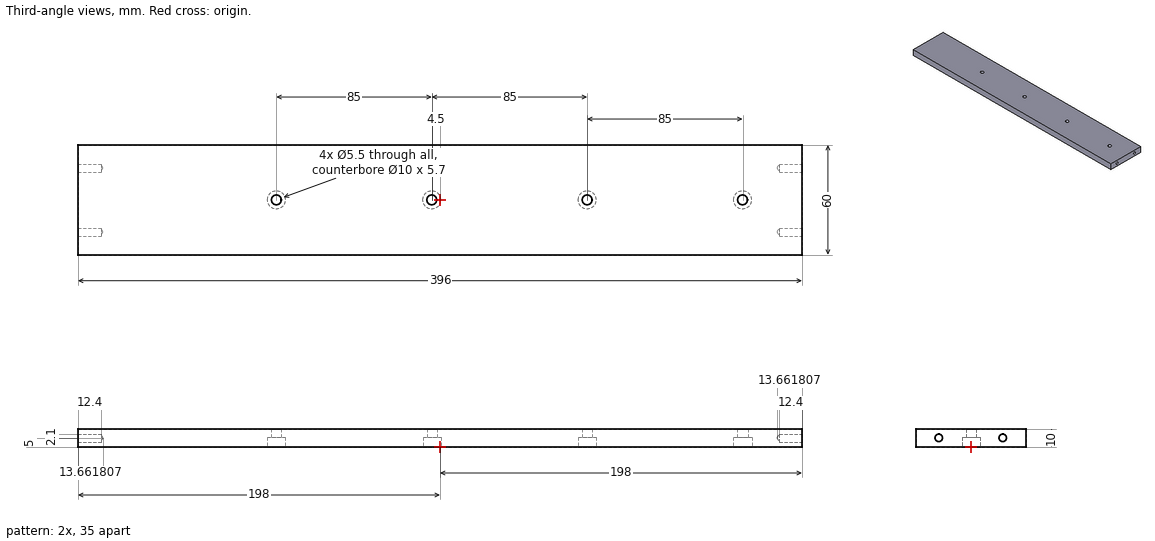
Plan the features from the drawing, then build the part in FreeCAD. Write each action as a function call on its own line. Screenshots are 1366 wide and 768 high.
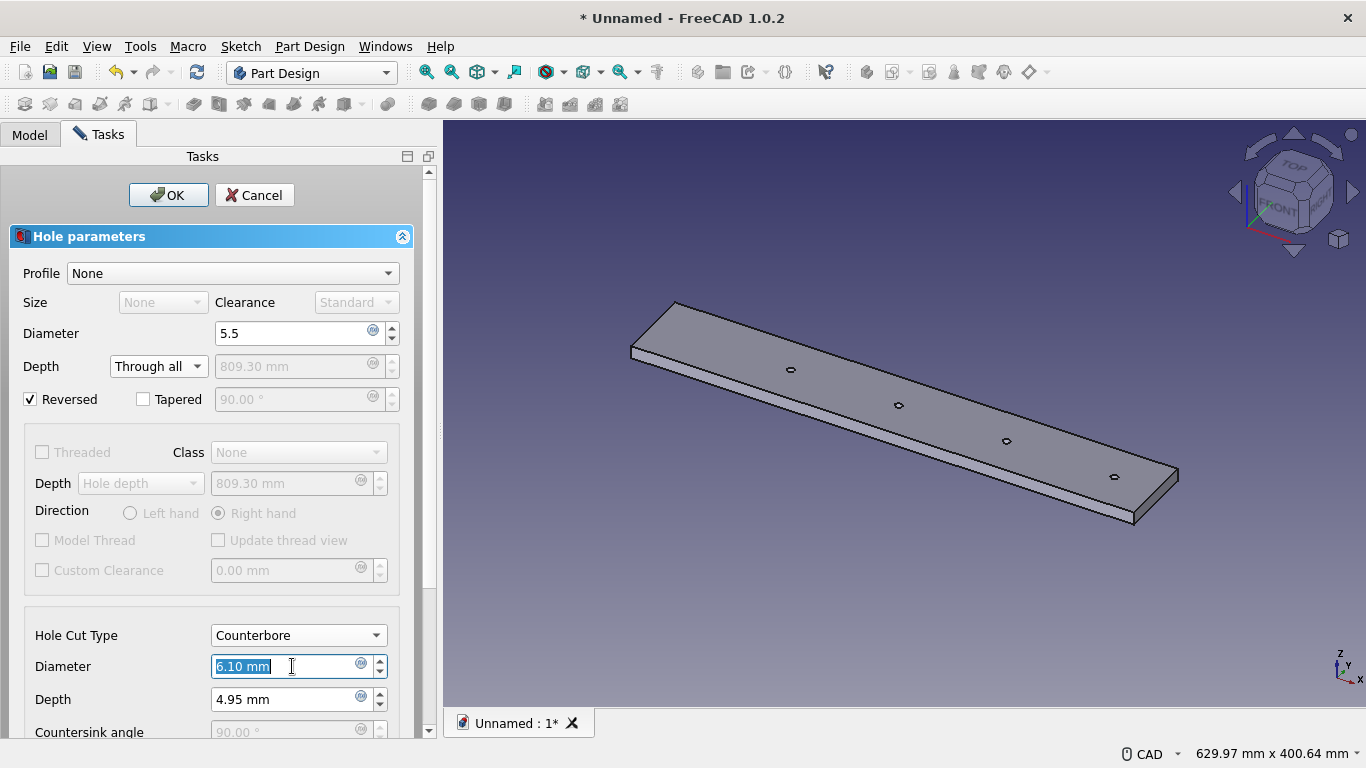
text(10)
key(Tab)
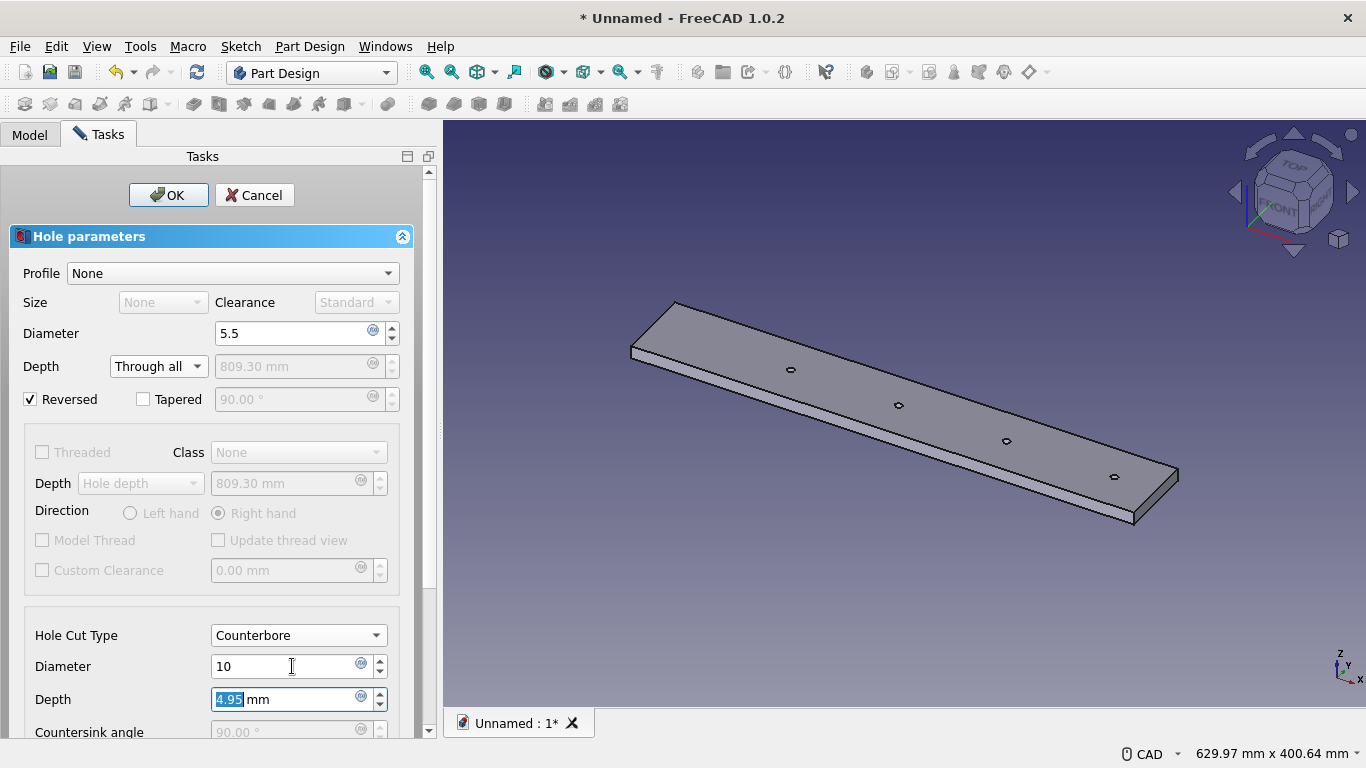
text(5.7)
key(Tab)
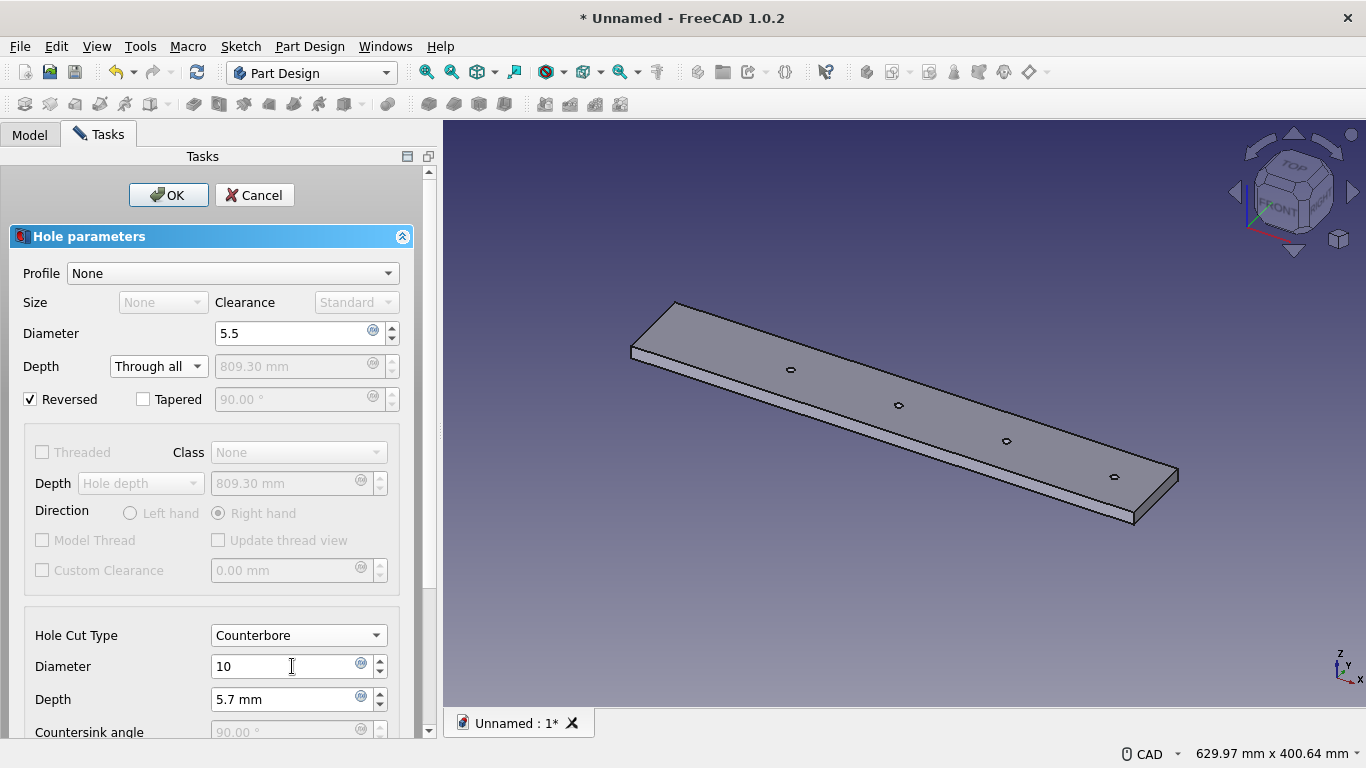
click(169, 195)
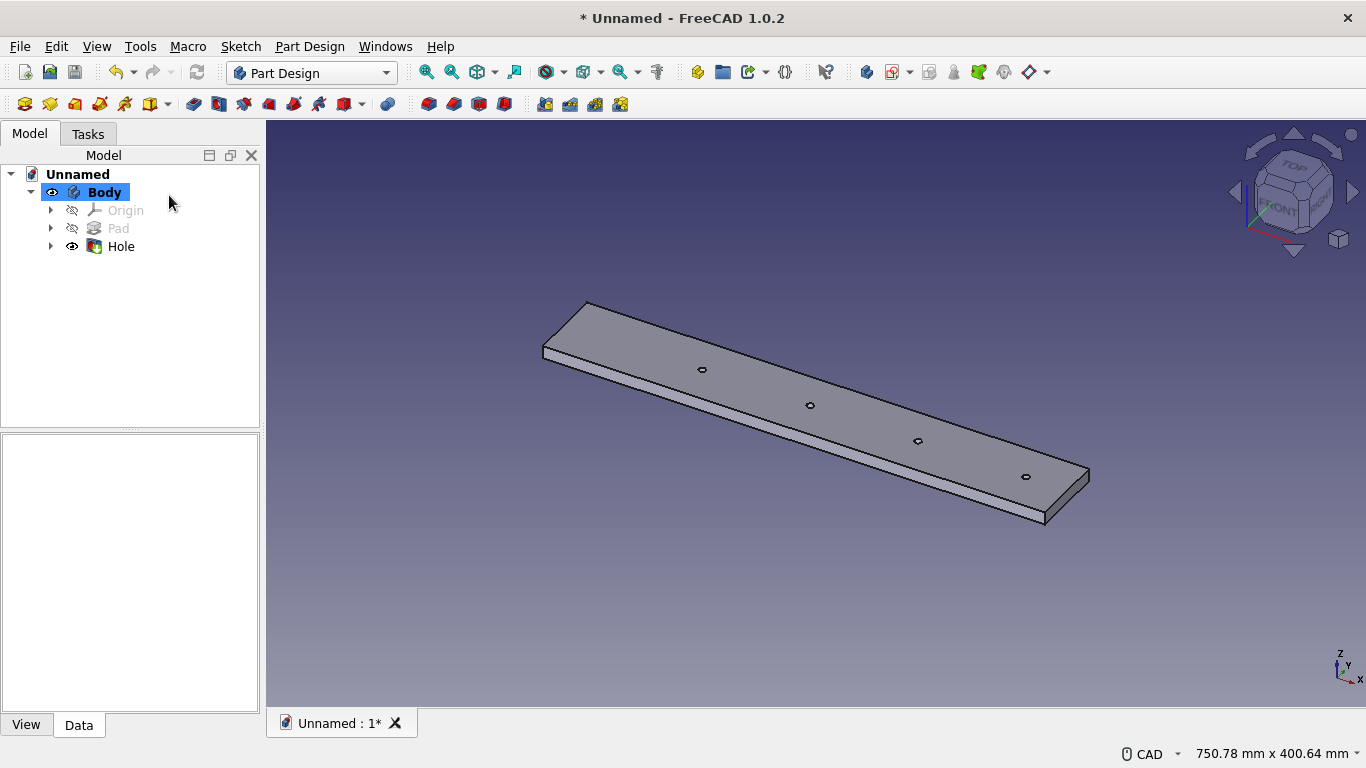
click(51, 210)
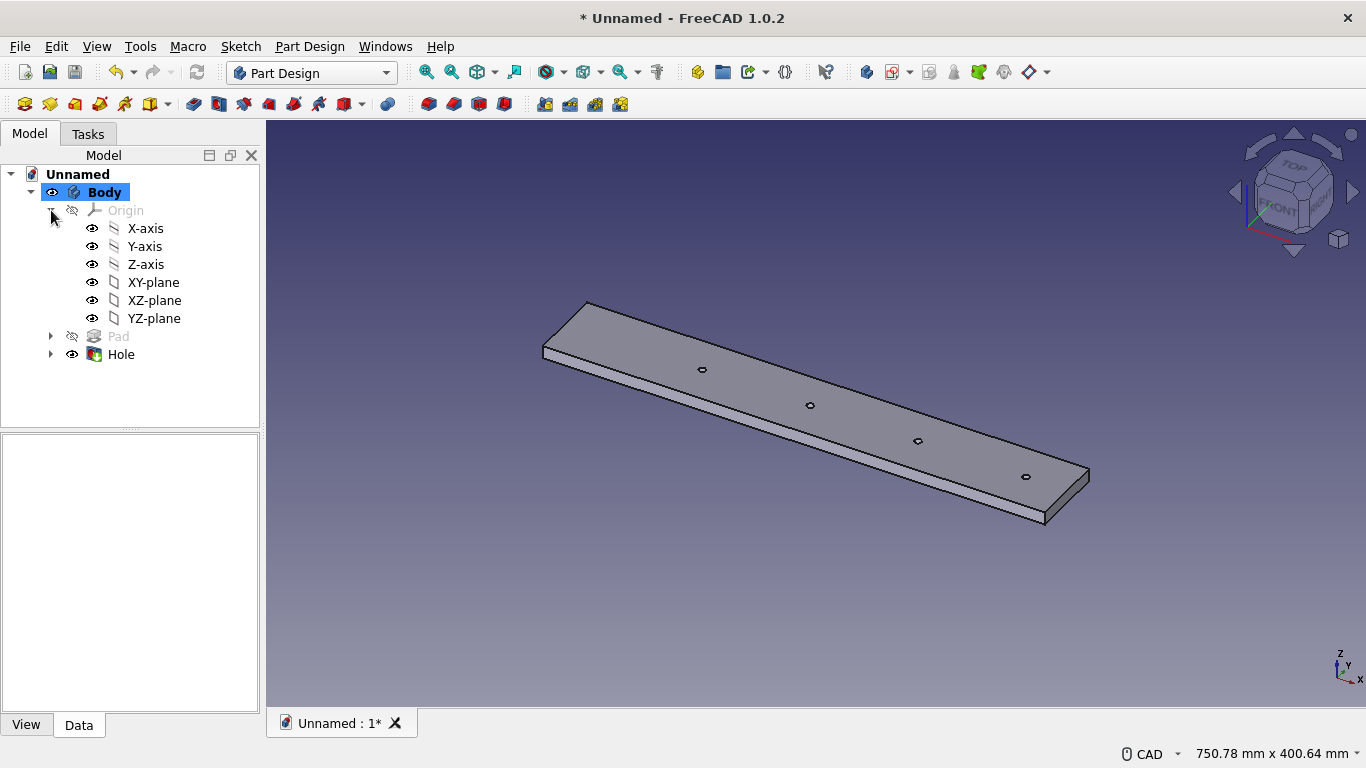
click(137, 300)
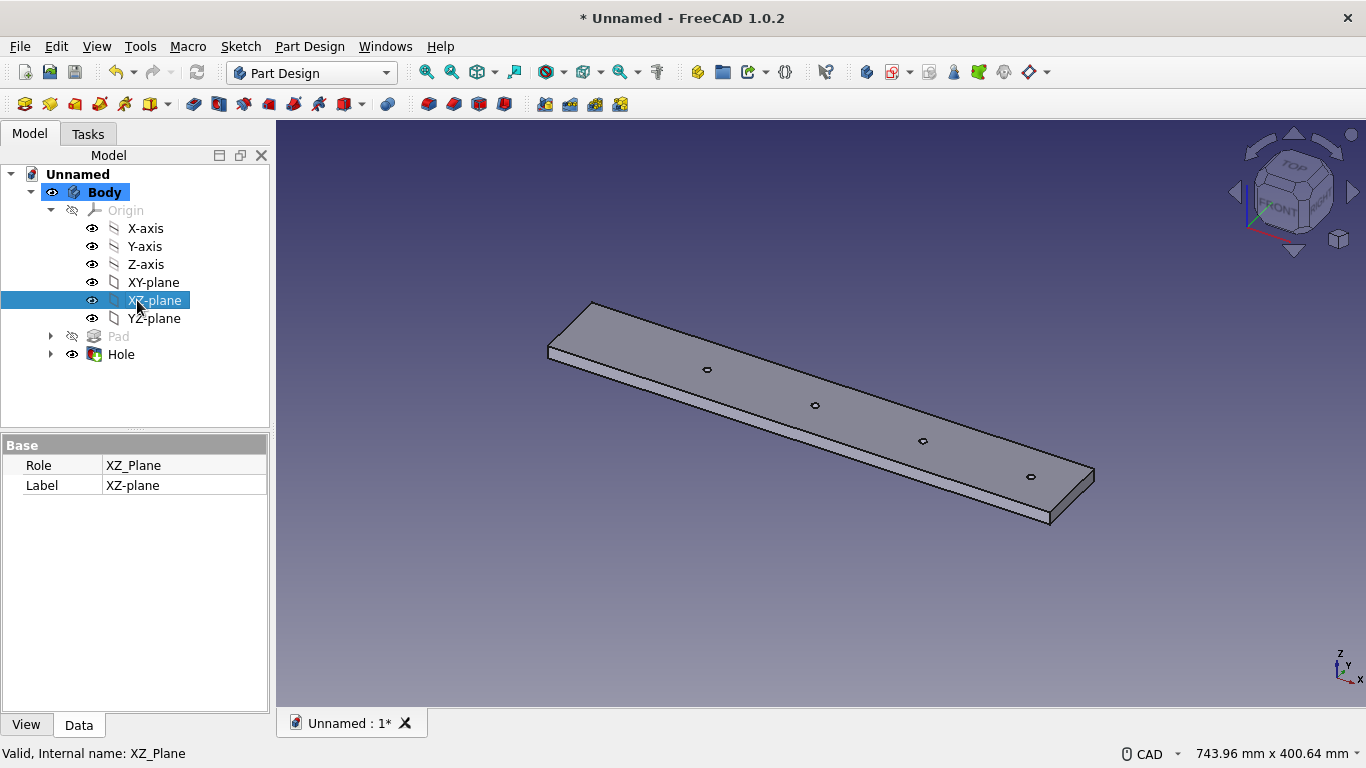
click(1028, 72)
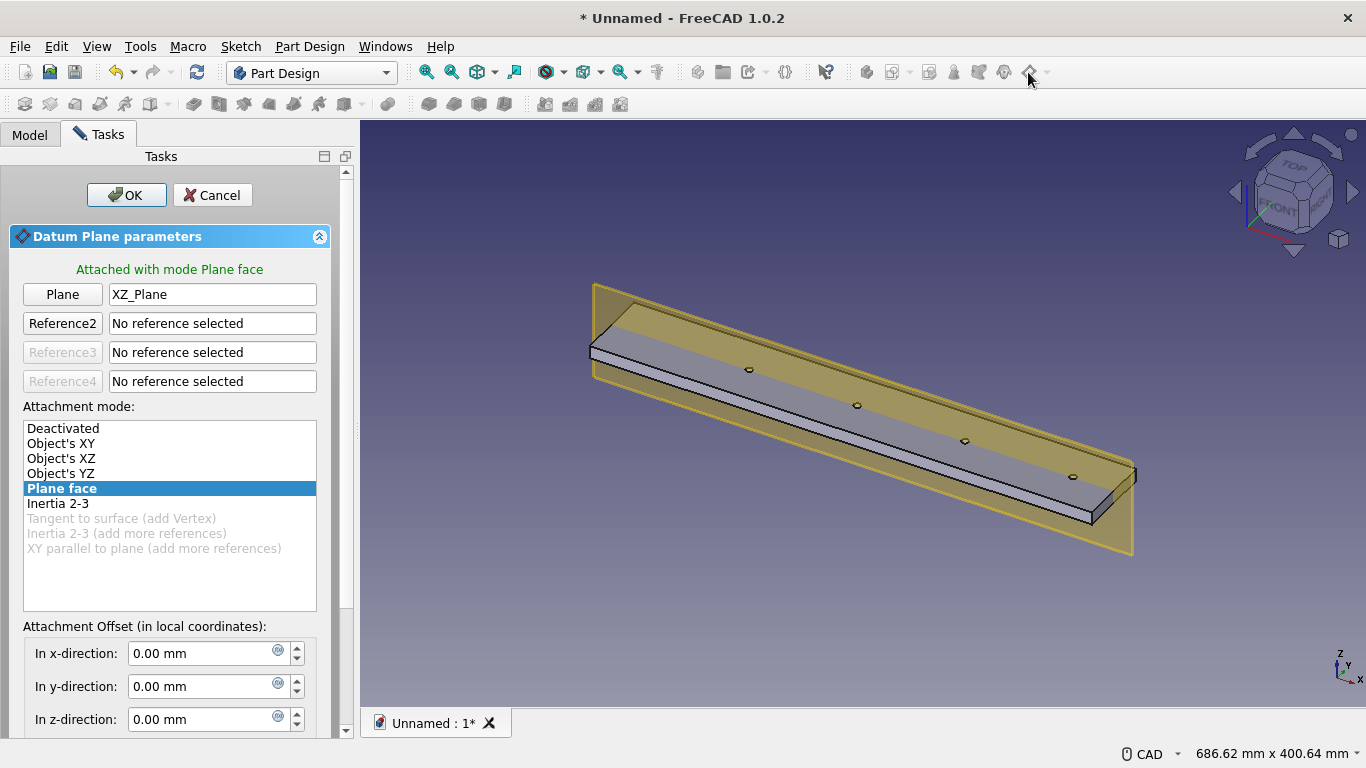
triple_click(210, 720)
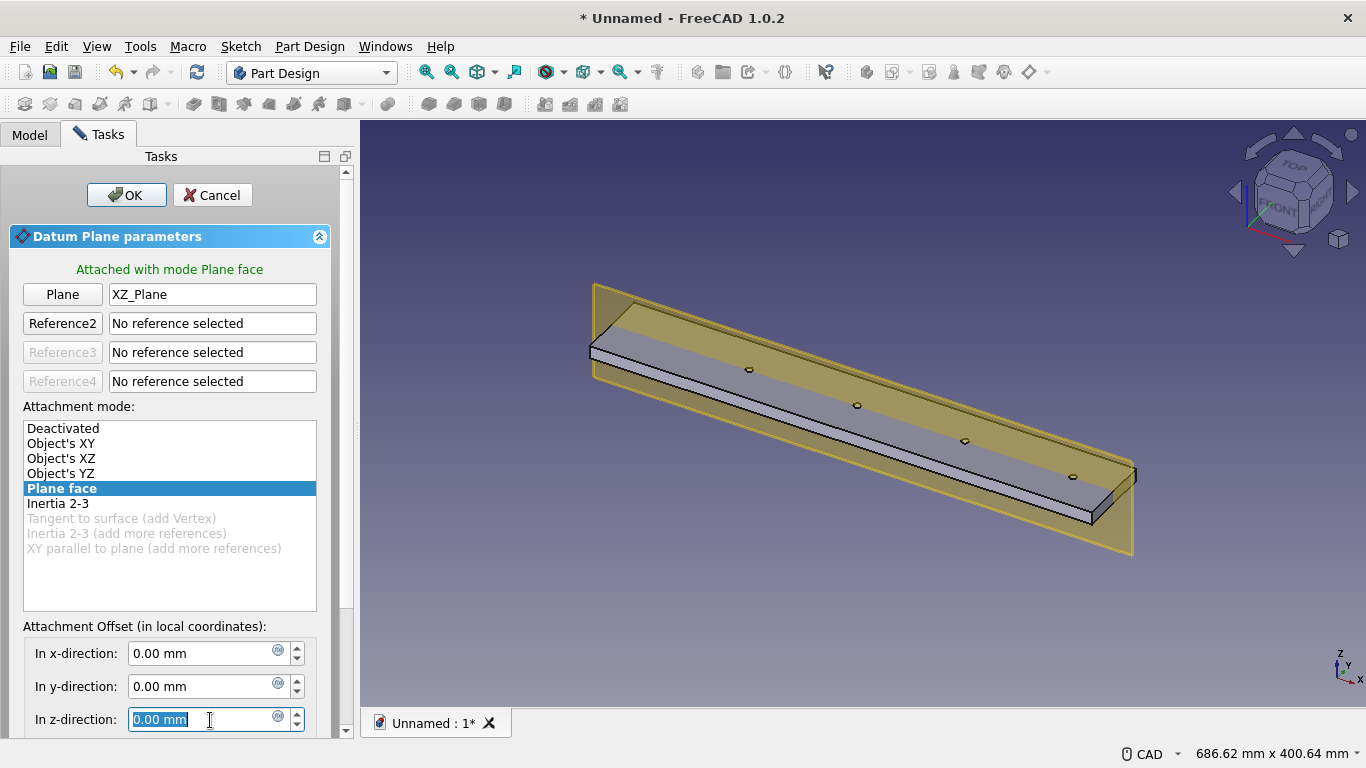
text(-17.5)
key(Tab)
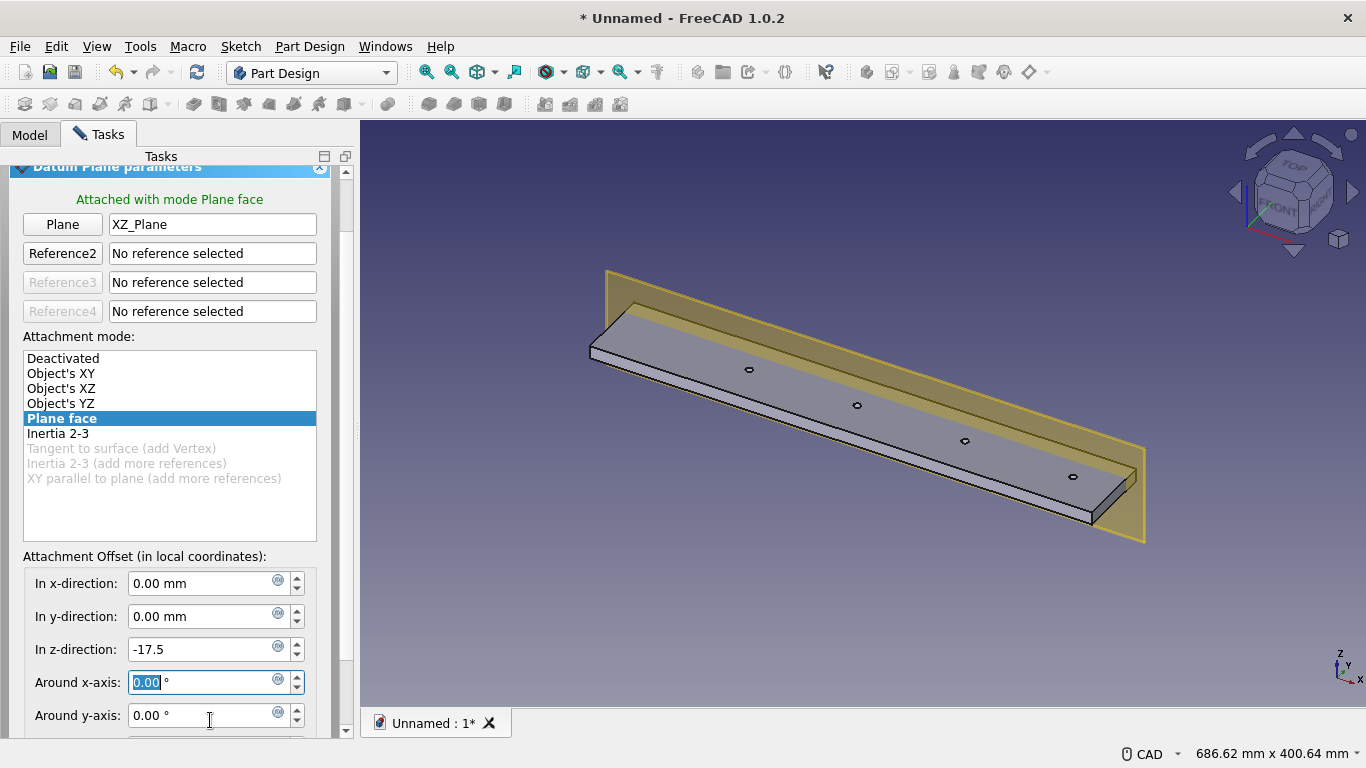
scroll(346, 452, up, 2)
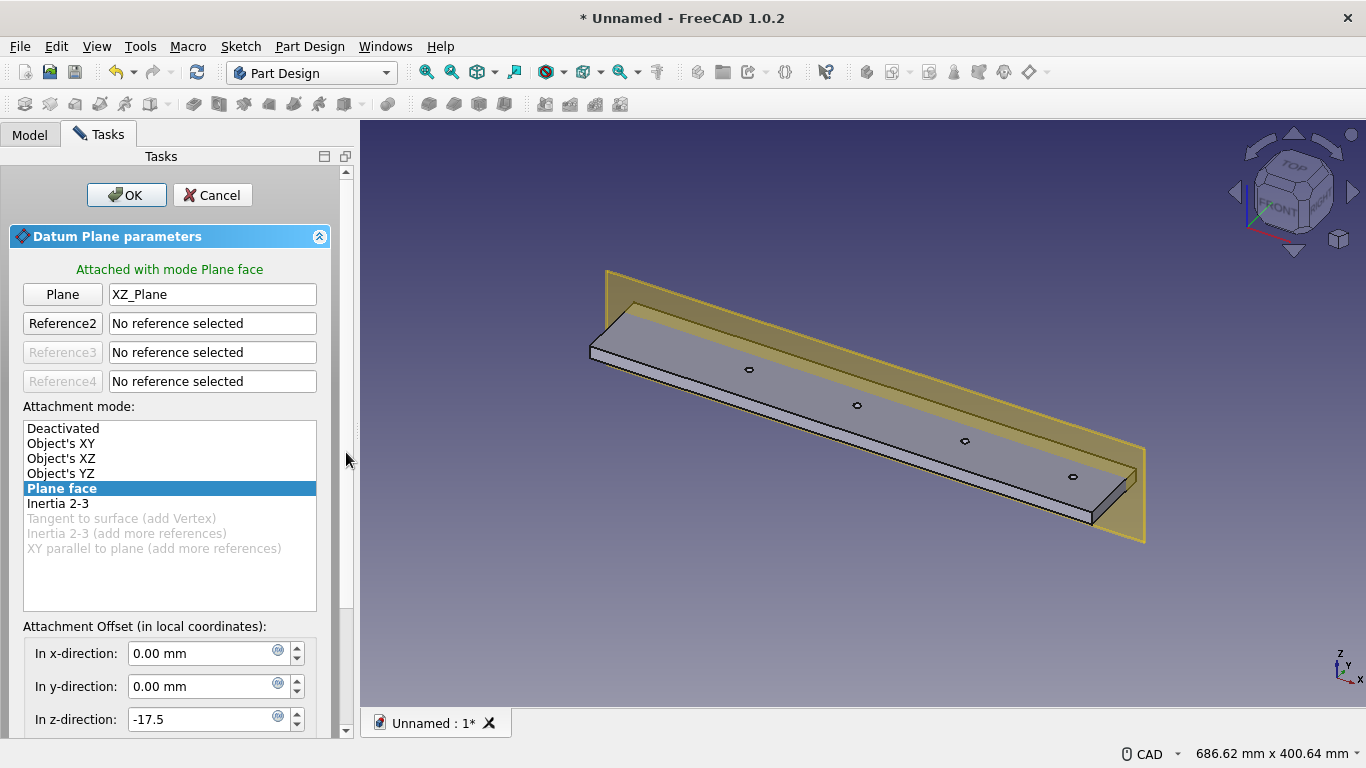
click(127, 195)